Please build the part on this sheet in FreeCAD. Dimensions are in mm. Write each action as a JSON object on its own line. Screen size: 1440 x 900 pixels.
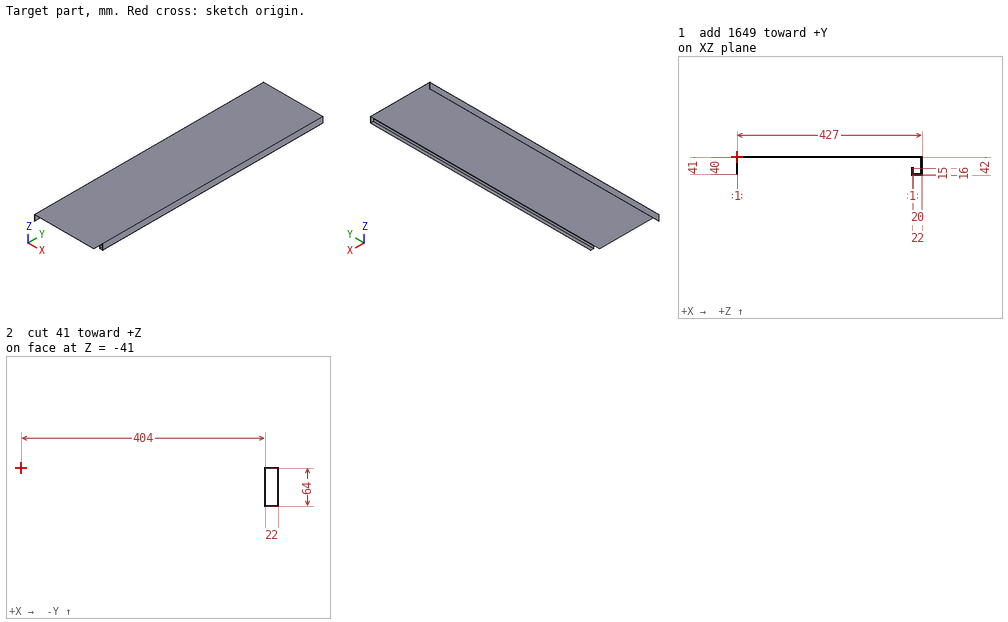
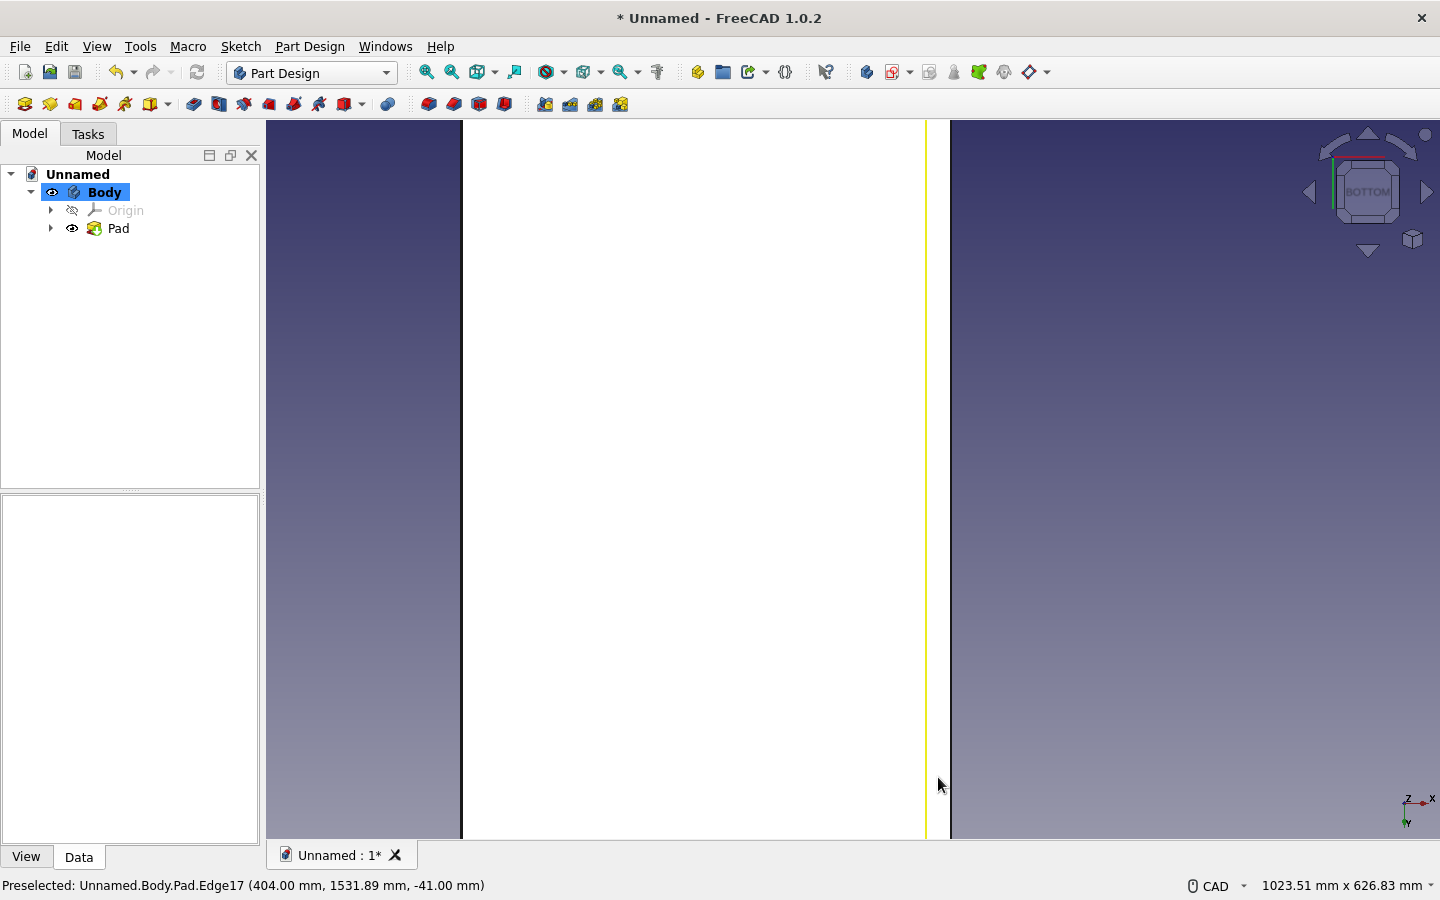
{"action": "left_click", "coordinate": [938, 776]}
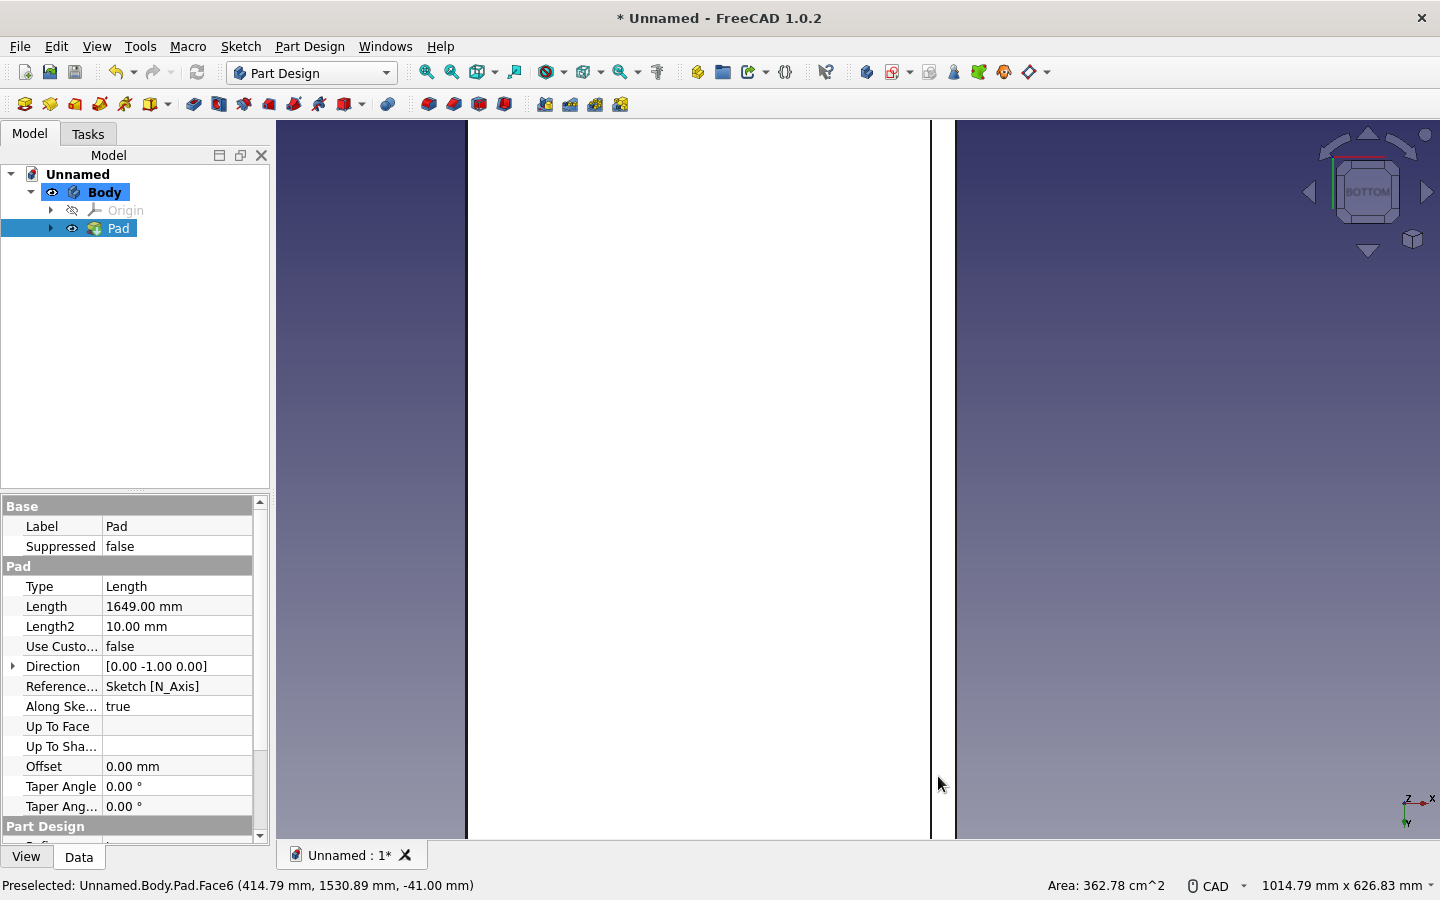
{"action": "left_click", "coordinate": [892, 72]}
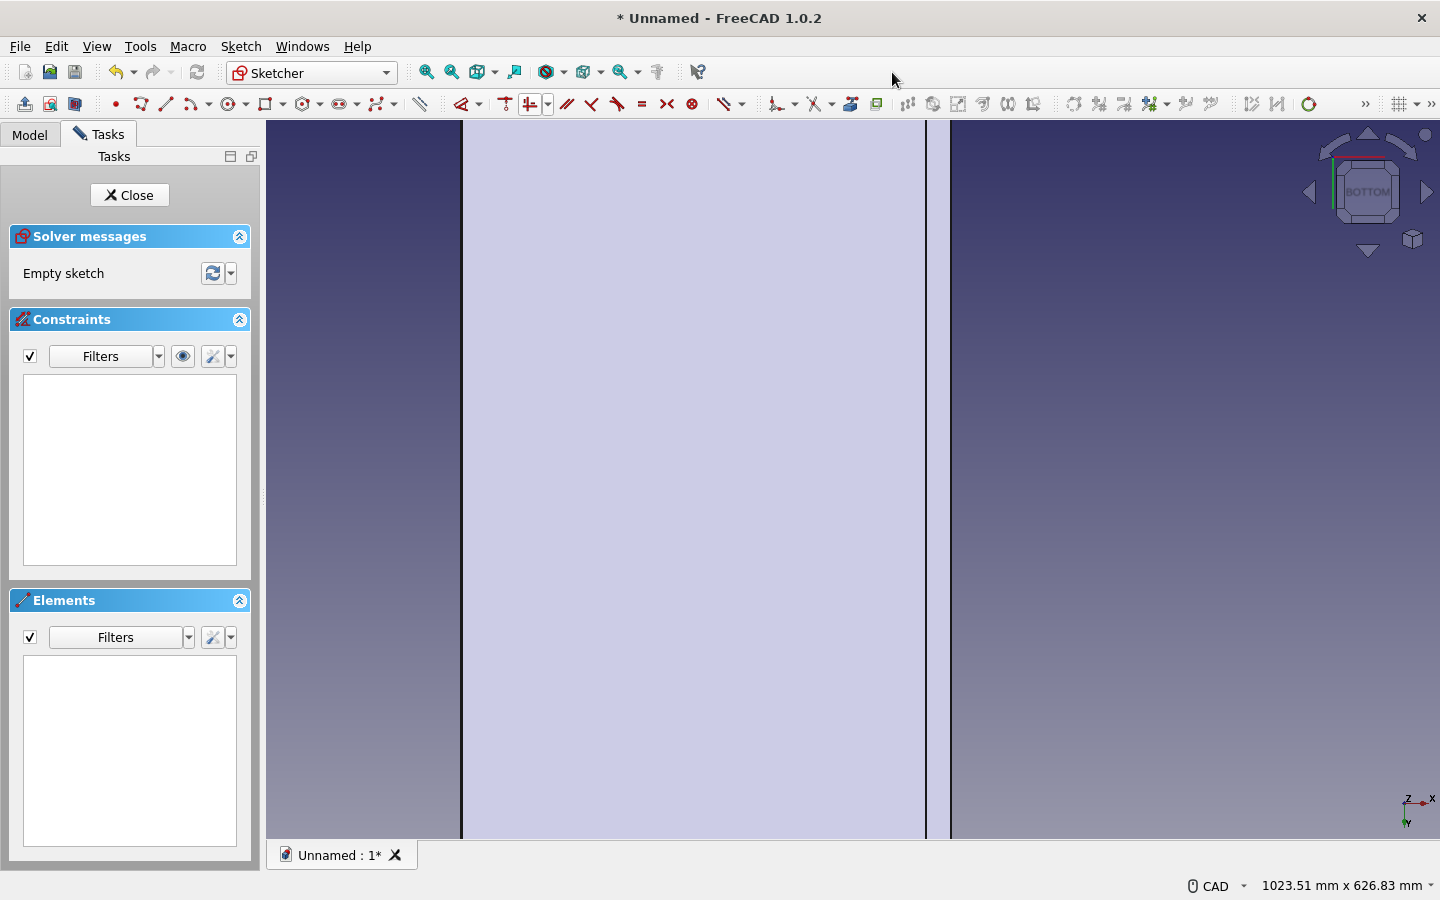
{"action": "scroll", "coordinate": [784, 480], "scroll_direction": "down", "scroll_amount": 5}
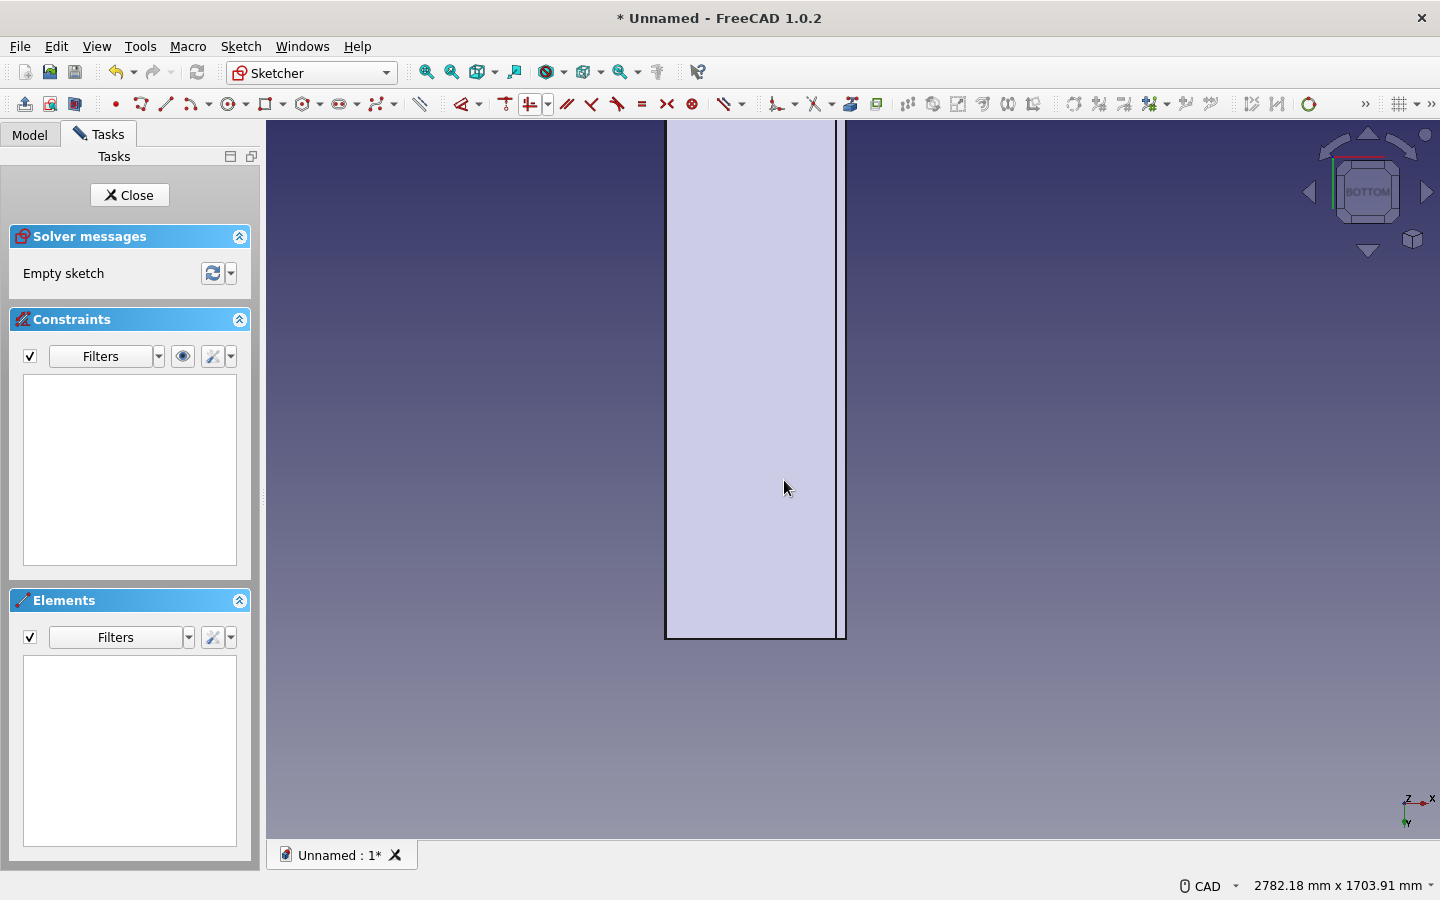
{"action": "scroll", "coordinate": [784, 480], "scroll_direction": "down", "scroll_amount": 5}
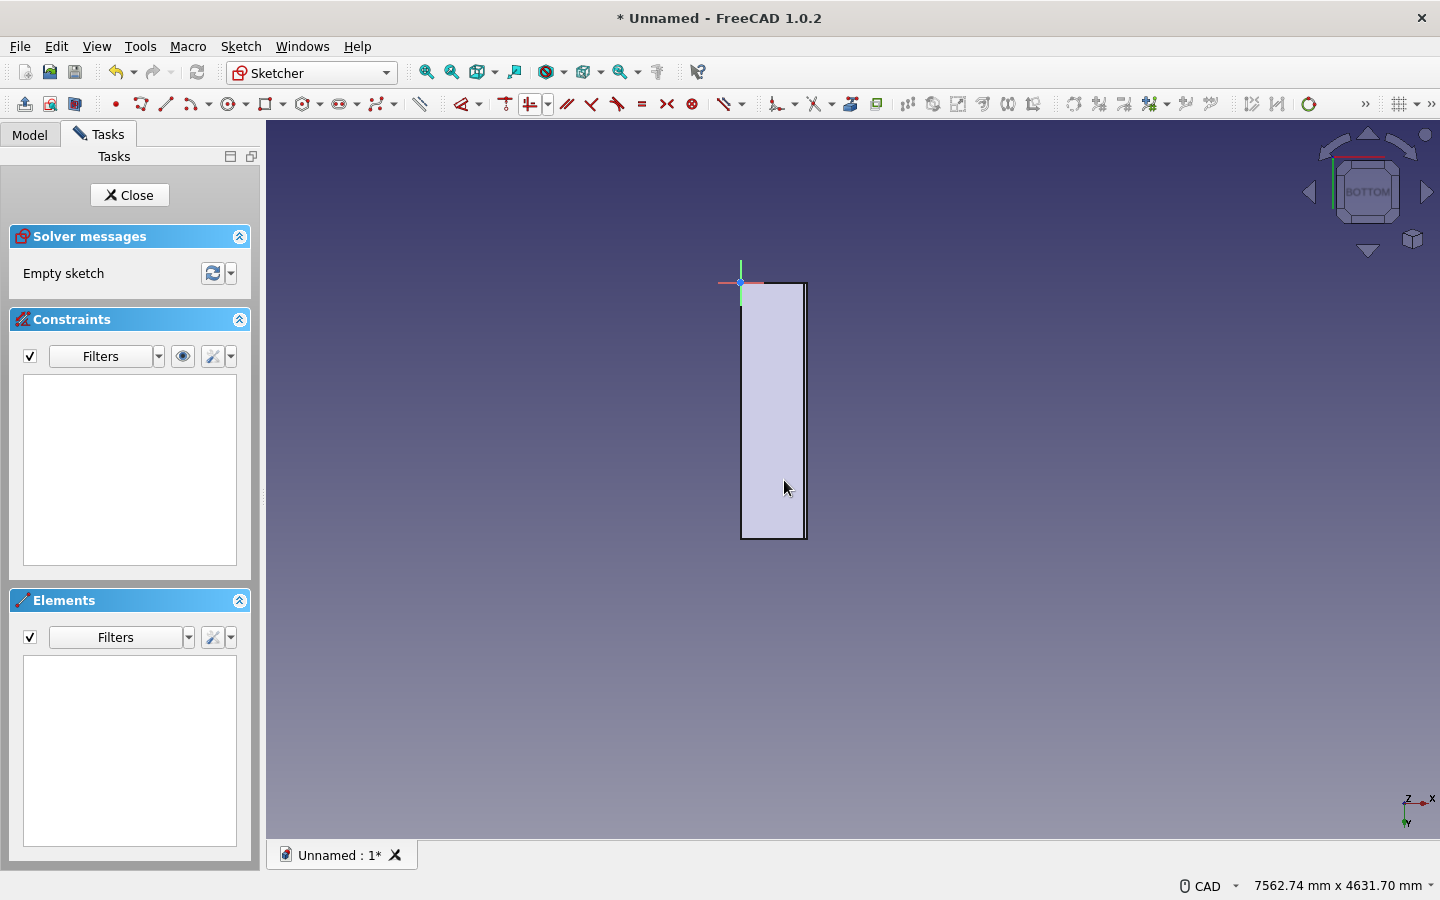
{"action": "scroll", "coordinate": [806, 278], "scroll_direction": "up", "scroll_amount": 15}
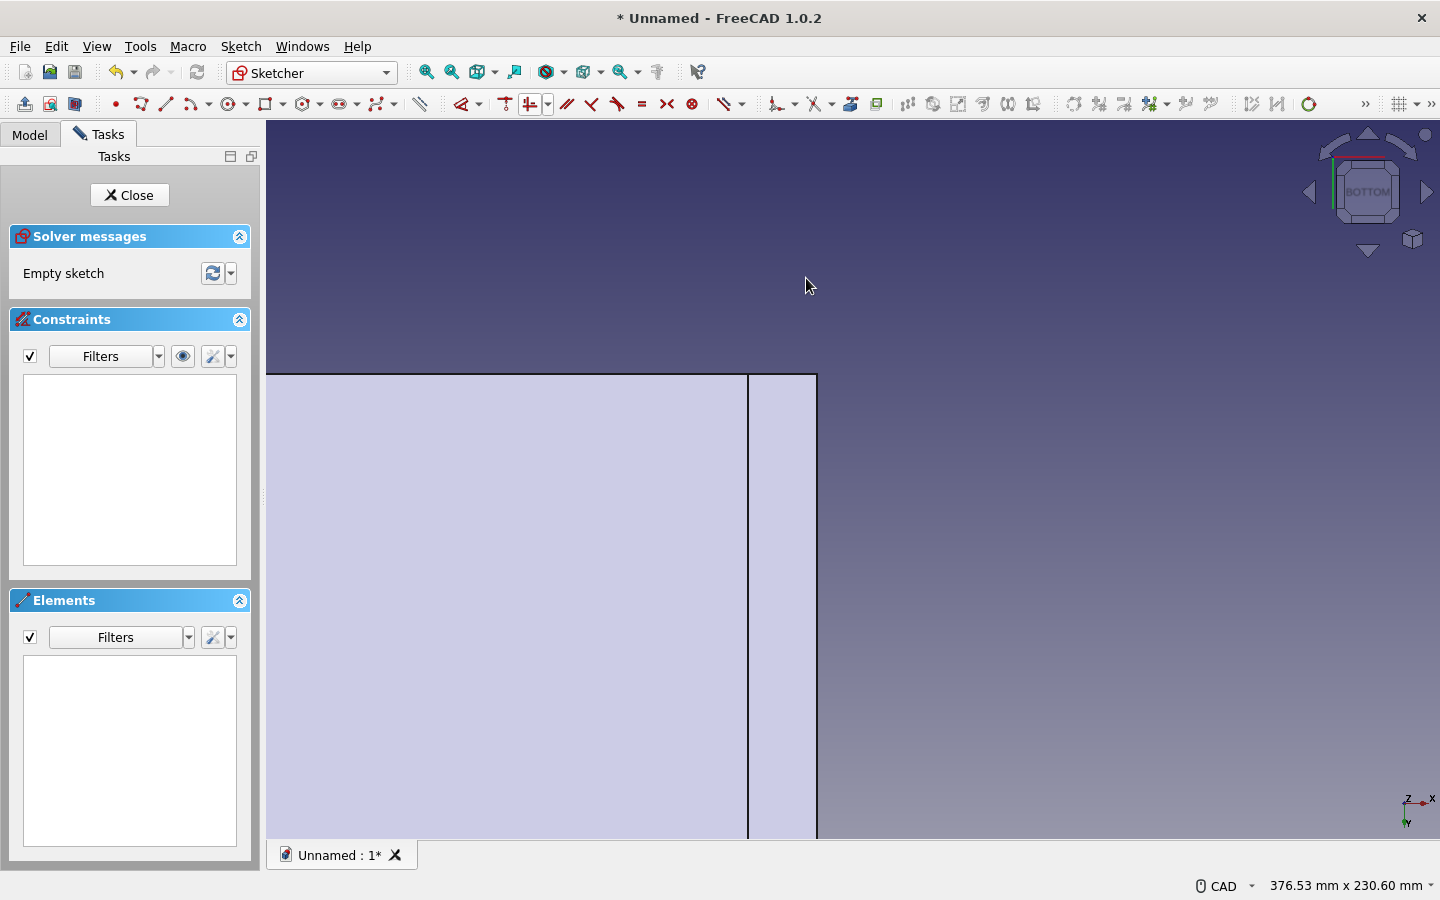
{"action": "scroll", "coordinate": [780, 469], "scroll_direction": "up", "scroll_amount": 4}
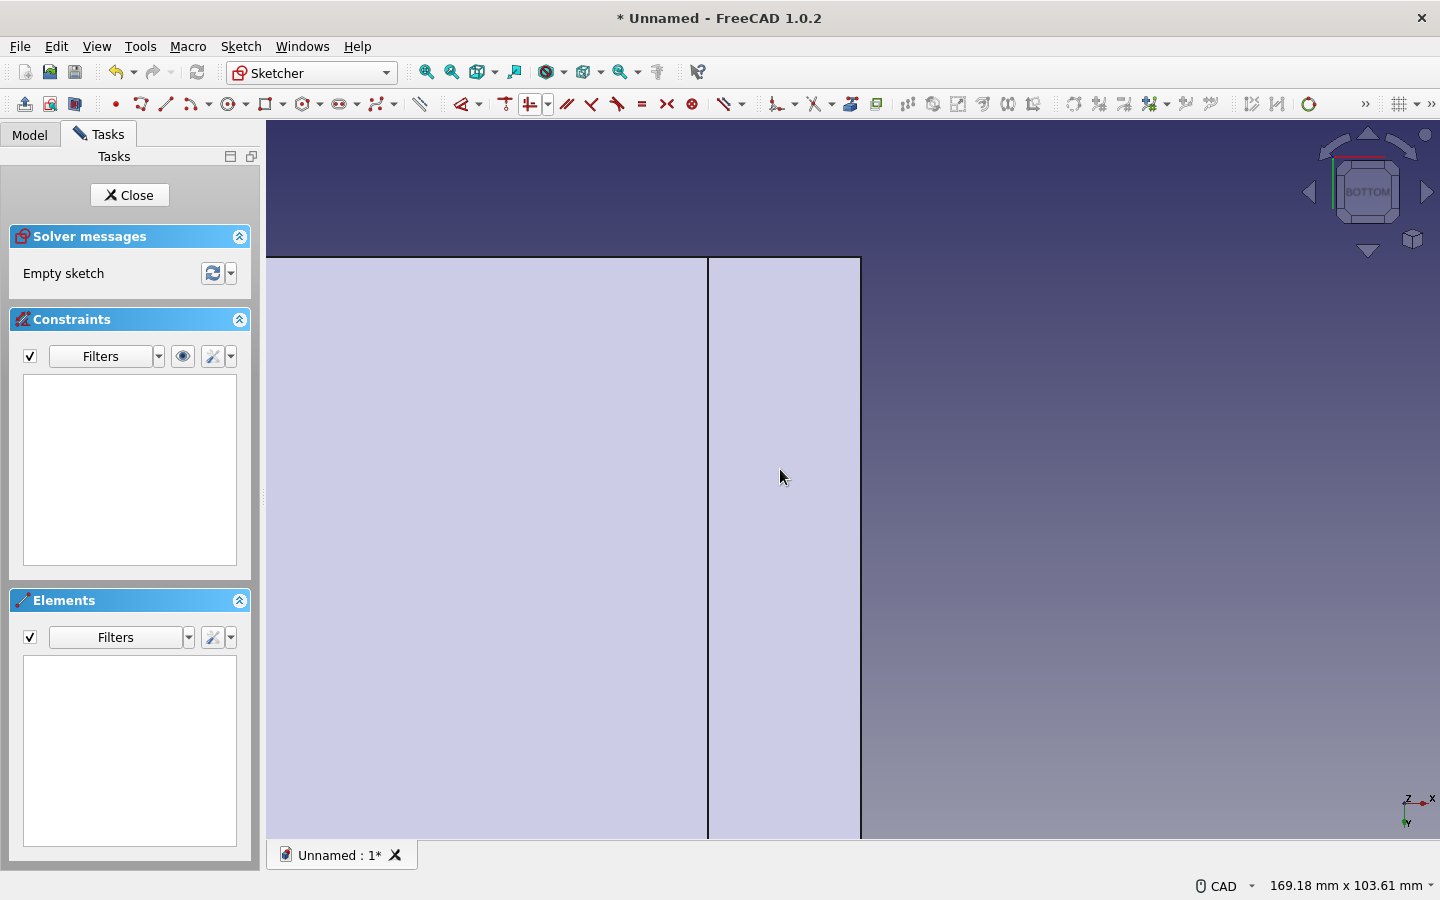
{"action": "left_click", "coordinate": [264, 104]}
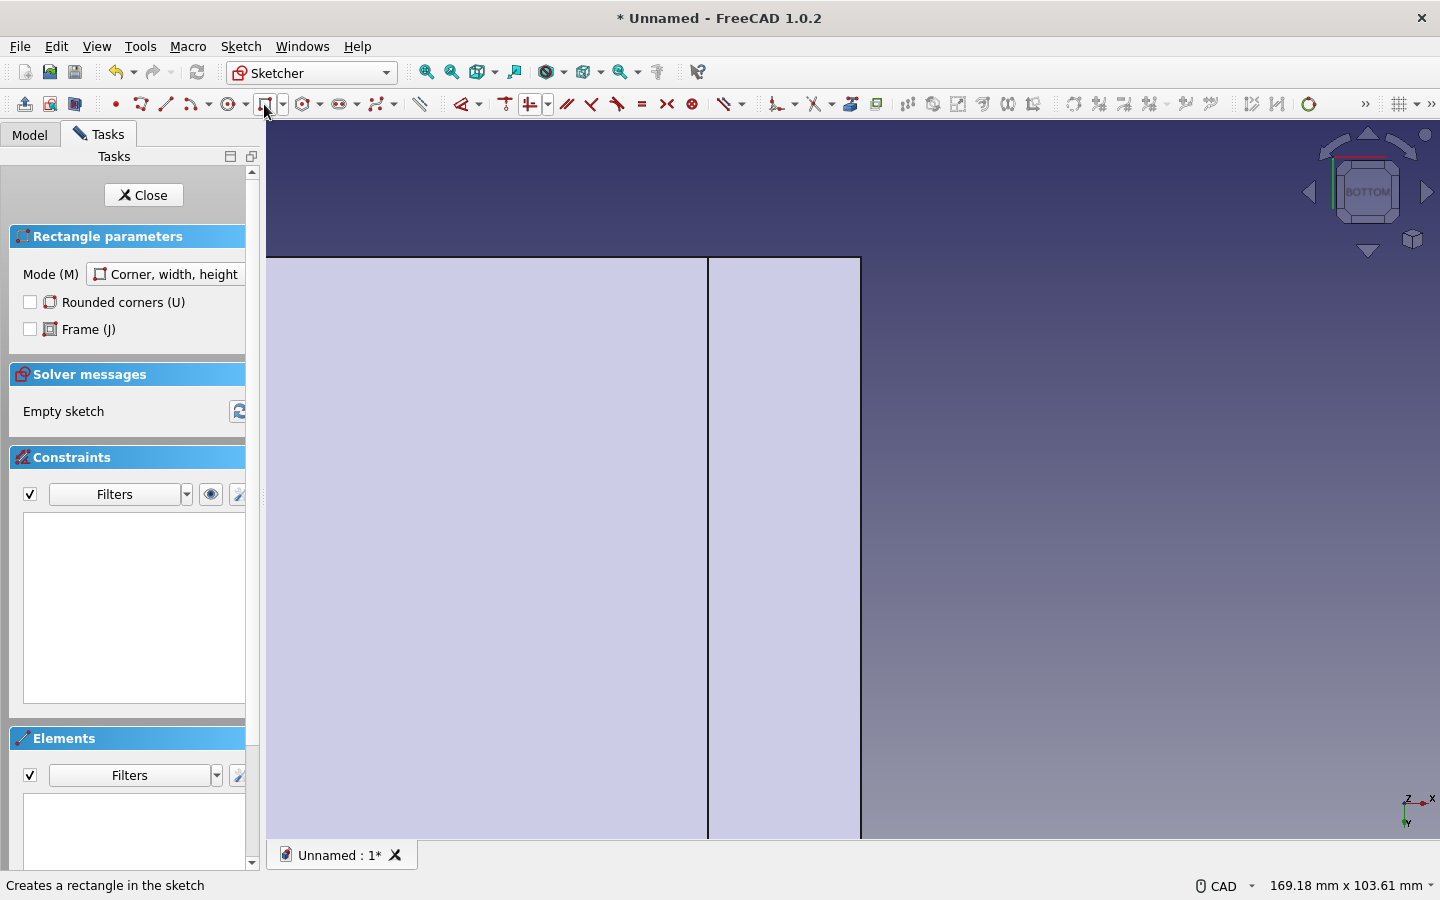
{"action": "left_click", "coordinate": [708, 257]}
{"action": "left_click", "coordinate": [861, 701]}
{"action": "key", "text": "Escape"}